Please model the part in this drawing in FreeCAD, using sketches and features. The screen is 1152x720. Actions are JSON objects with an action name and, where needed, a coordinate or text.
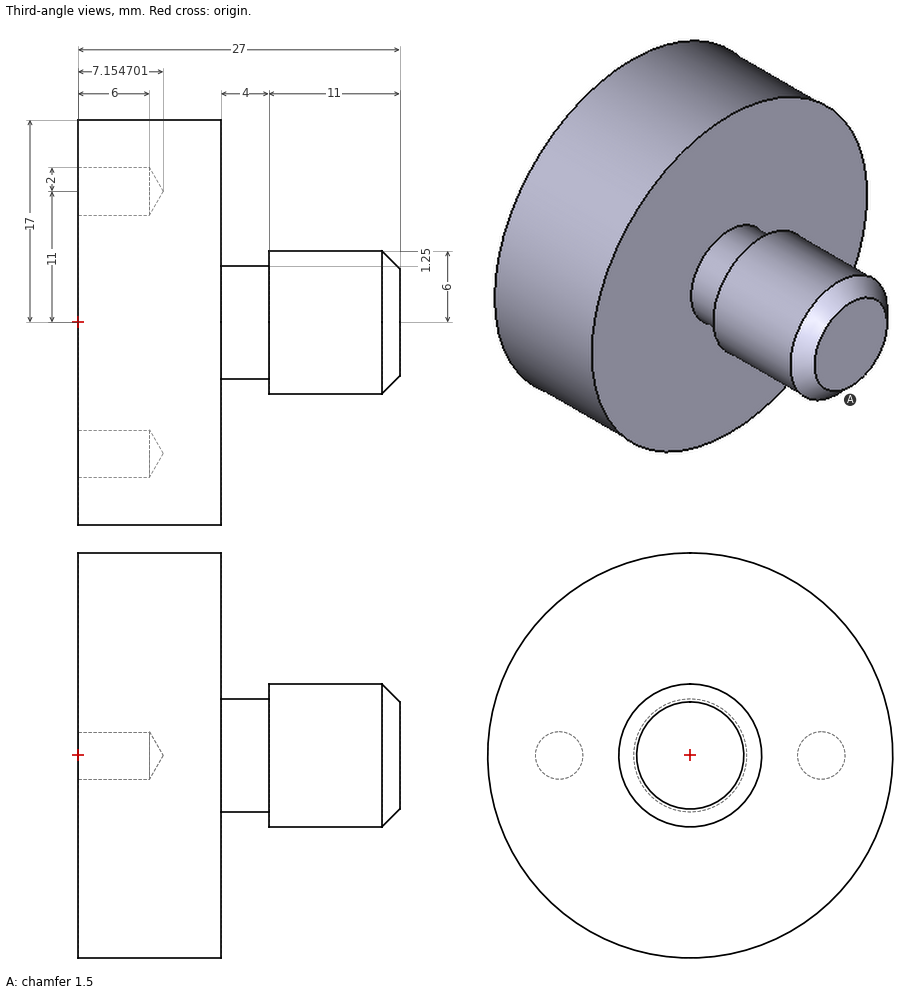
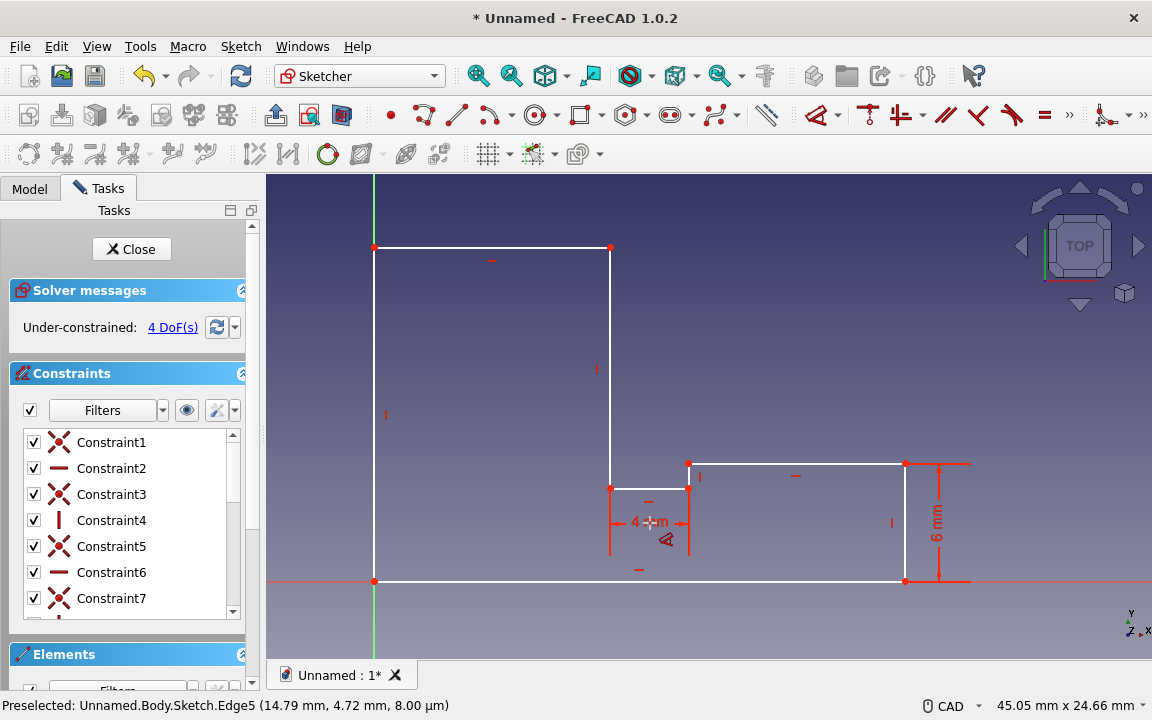
{"action": "left_click", "coordinate": [533, 582]}
{"action": "left_click", "coordinate": [640, 616]}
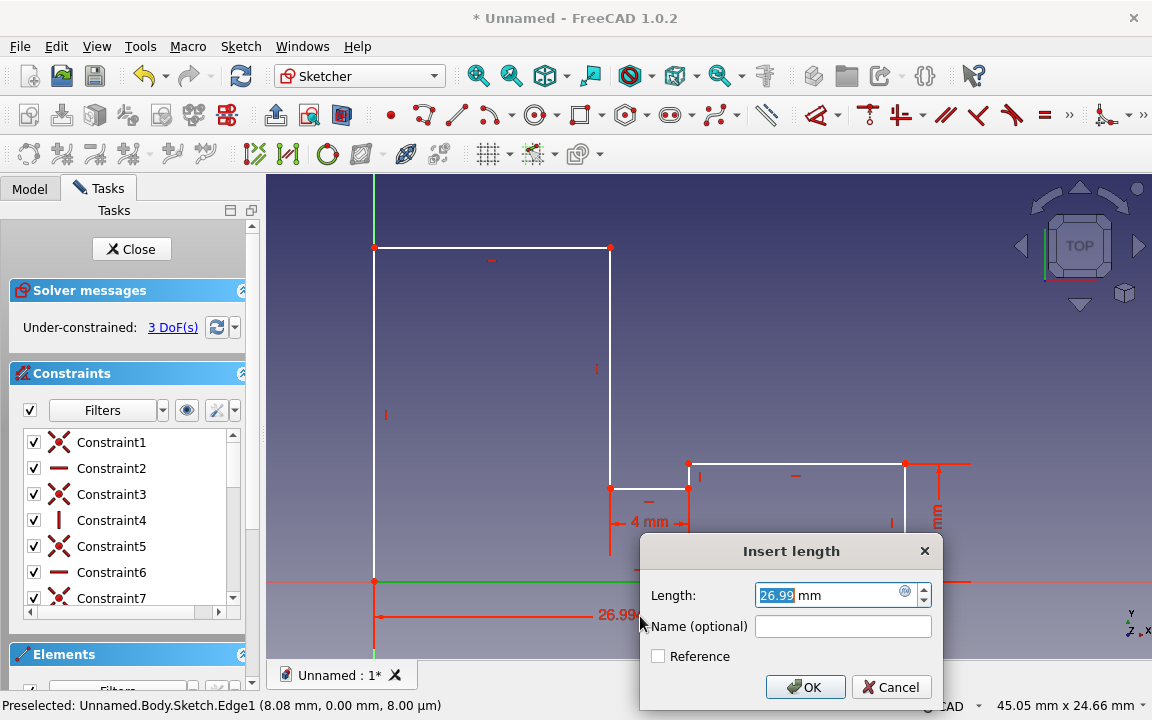
{"action": "type", "text": "27"}
{"action": "key", "text": "Return"}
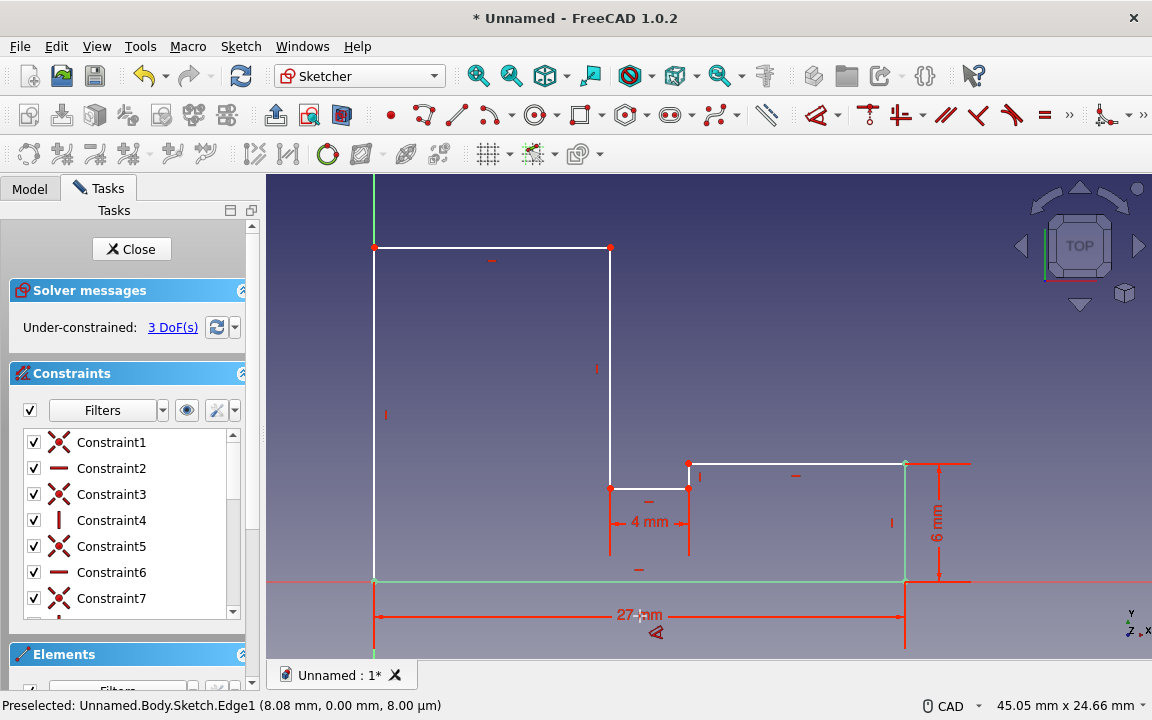
{"action": "left_click", "coordinate": [840, 464]}
{"action": "left_click", "coordinate": [797, 498]}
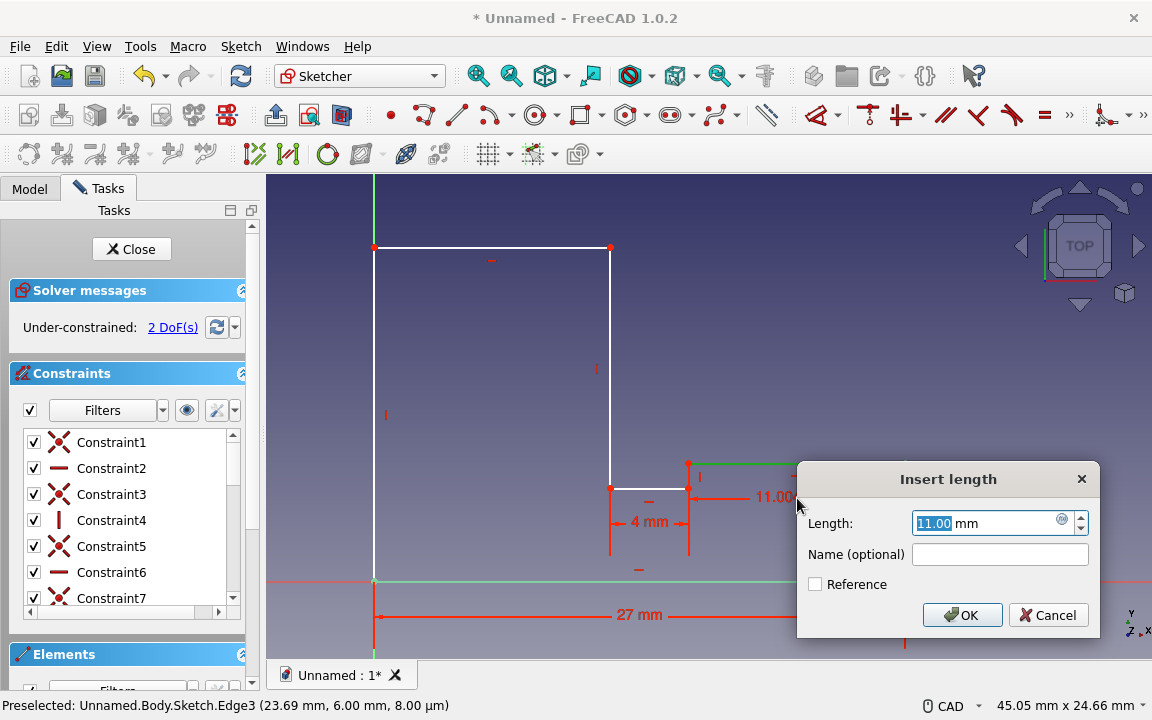
{"action": "type", "text": "11"}
{"action": "key", "text": "Return"}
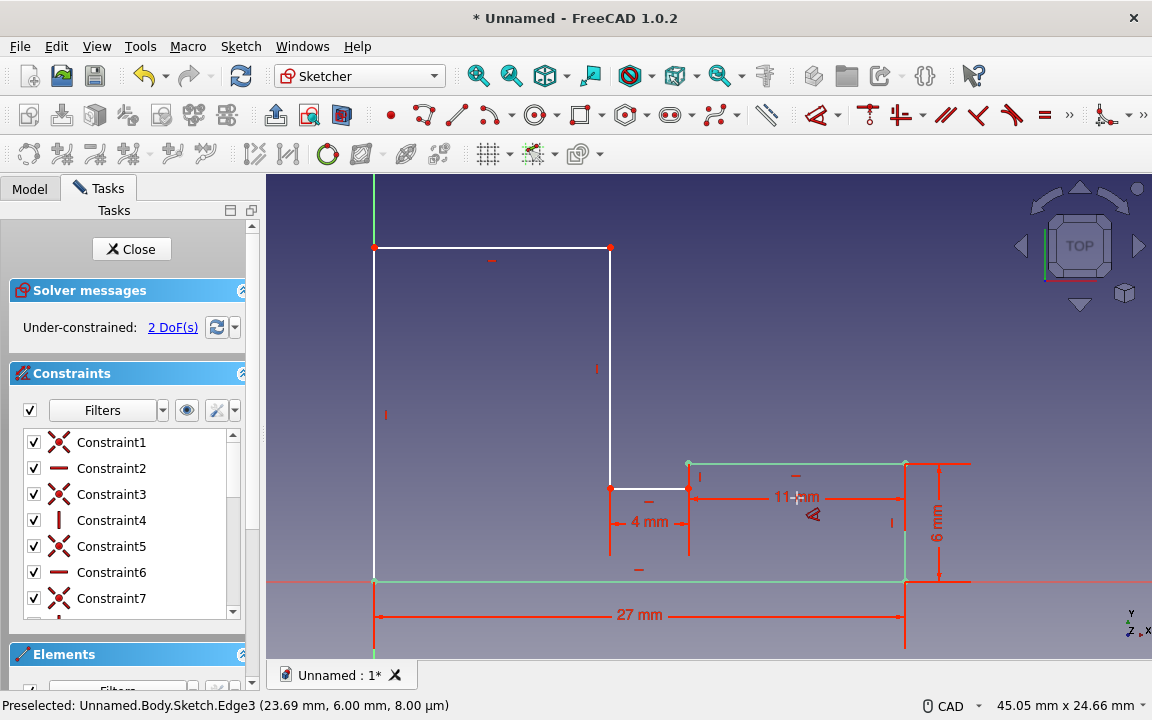
{"action": "left_click", "coordinate": [374, 348]}
{"action": "left_click", "coordinate": [340, 415]}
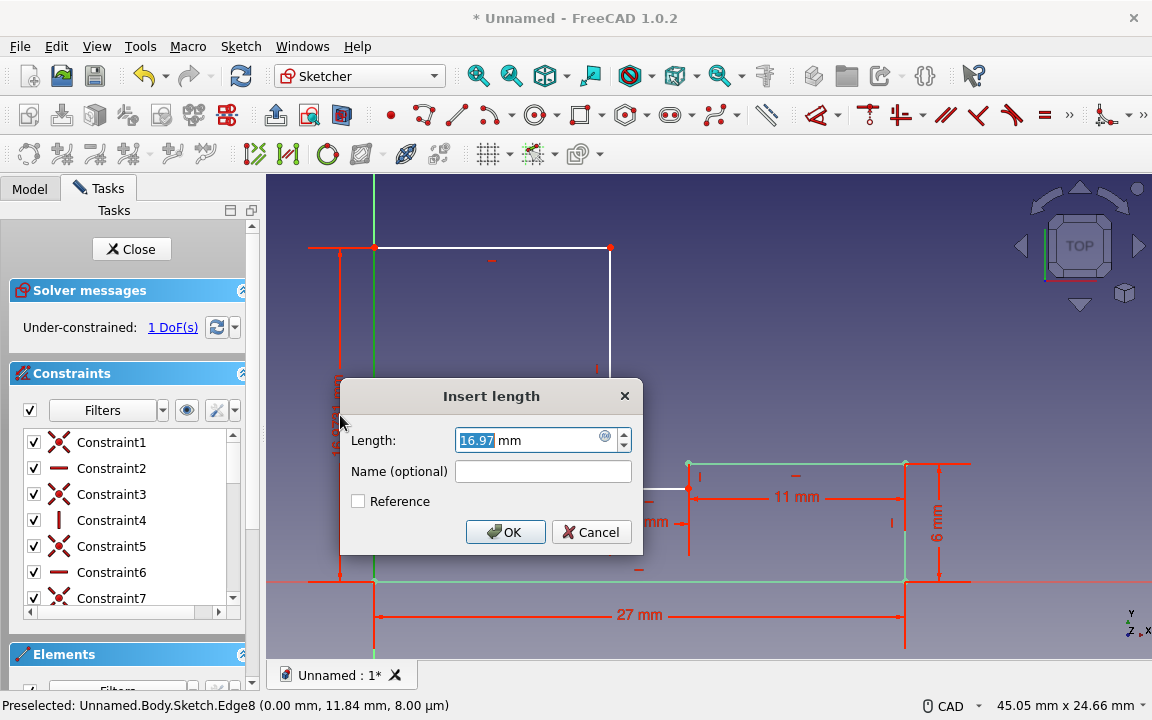
{"action": "type", "text": "17"}
{"action": "key", "text": "Return"}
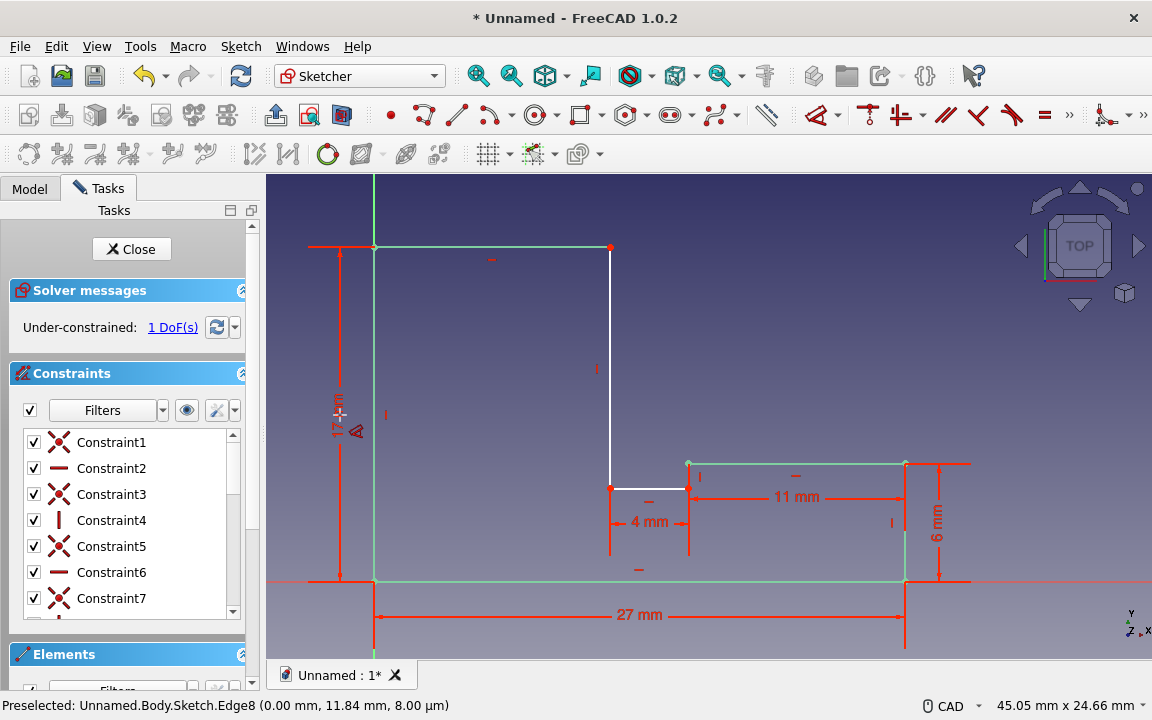
{"action": "scroll", "coordinate": [689, 474], "scroll_direction": "up", "scroll_amount": 3}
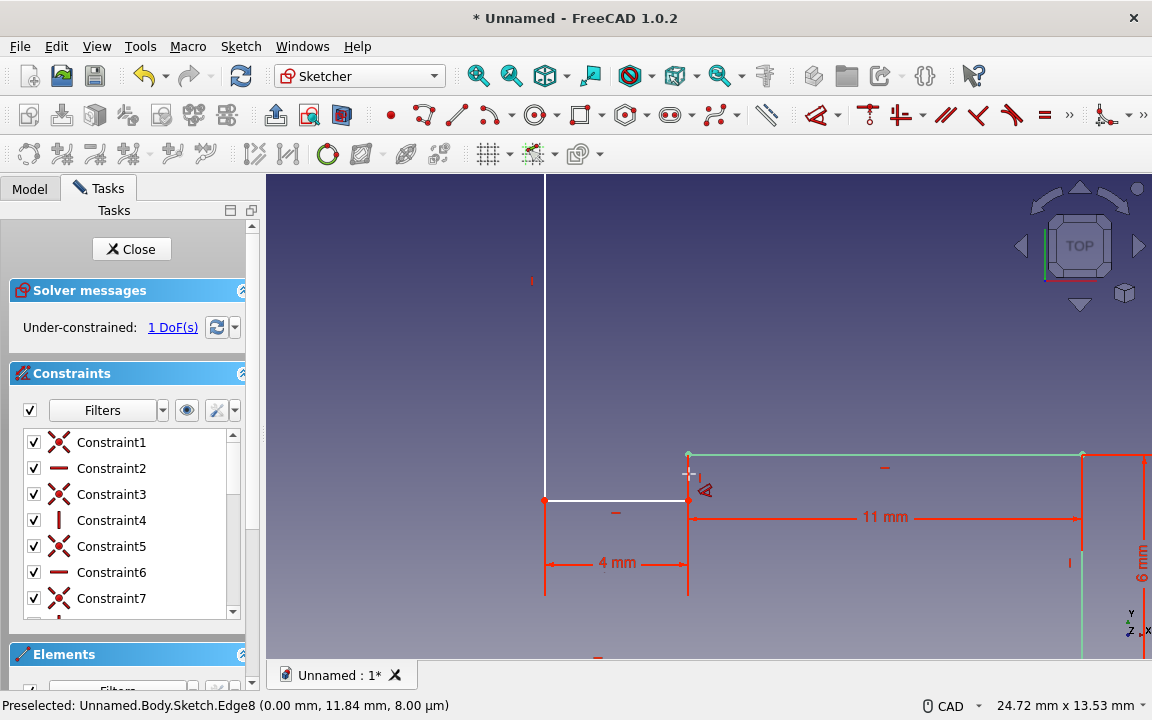
{"action": "left_click", "coordinate": [688, 473]}
{"action": "left_click", "coordinate": [722, 478]}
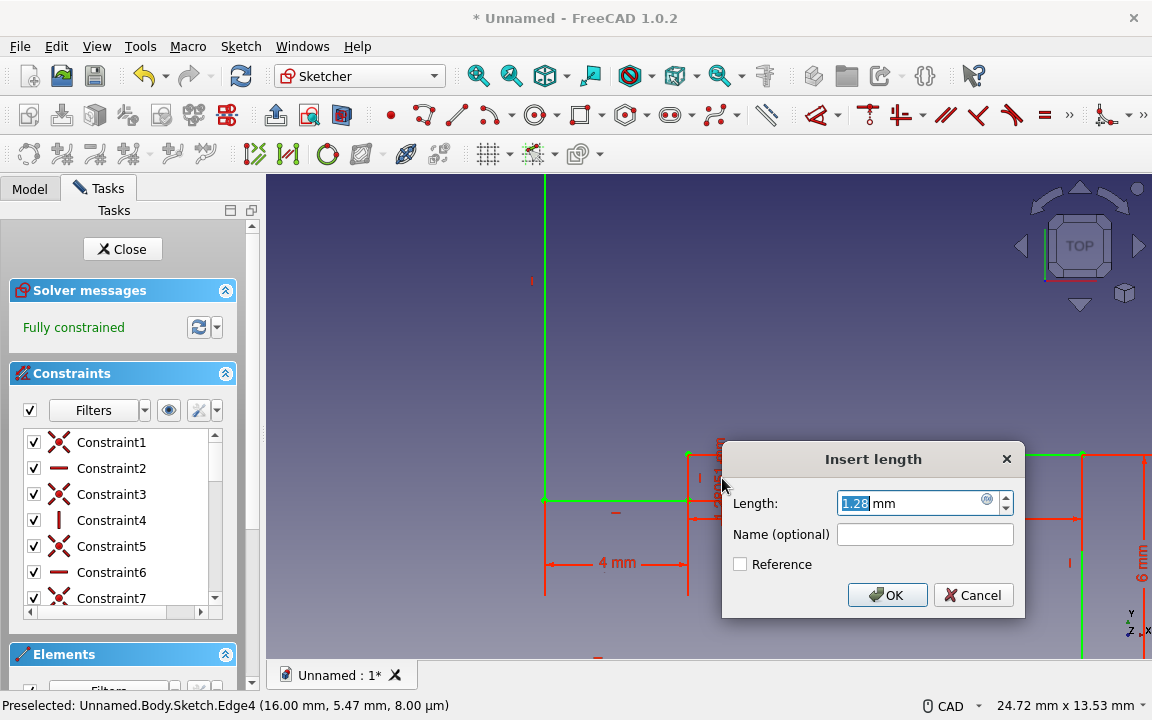
{"action": "type", "text": "1.25"}
{"action": "key", "text": "Return"}
{"action": "key", "text": "Escape"}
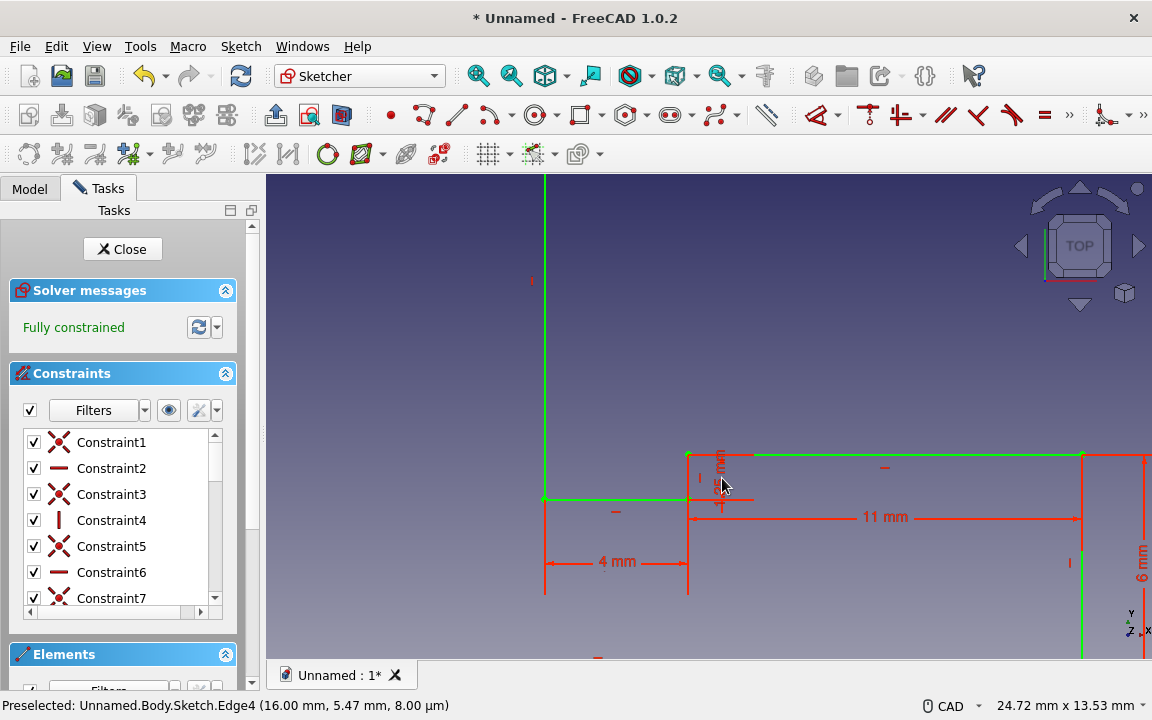
{"action": "left_click", "coordinate": [123, 249]}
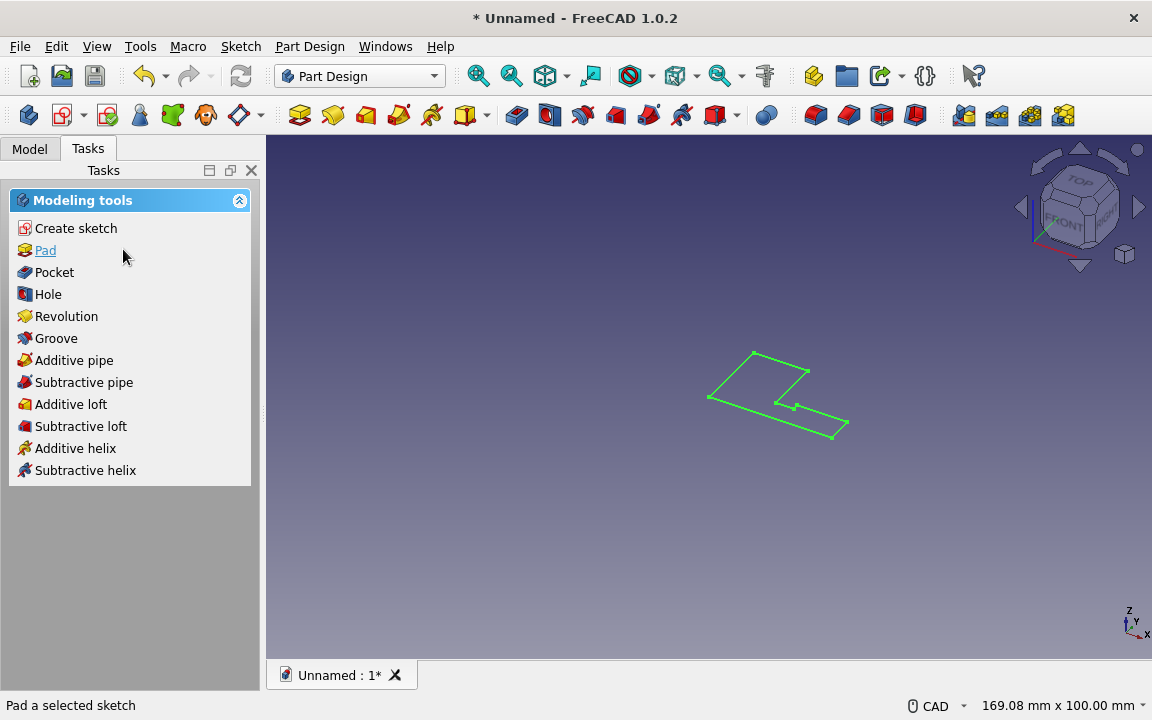
{"action": "left_click", "coordinate": [333, 116]}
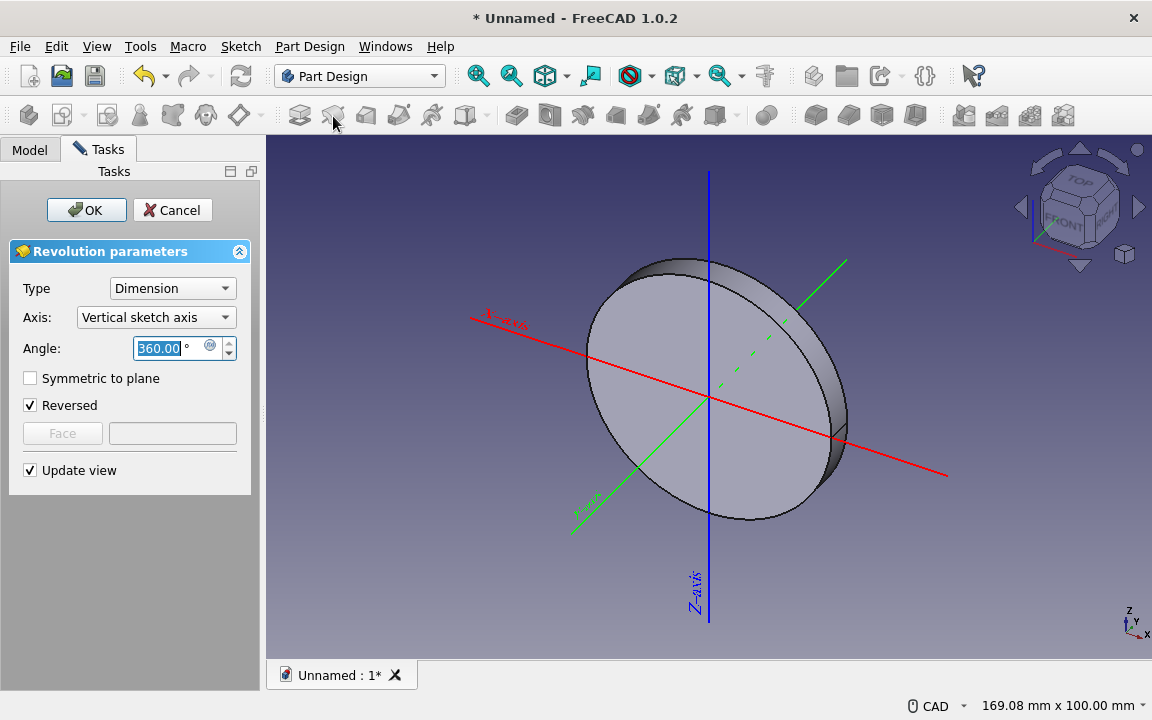
{"action": "left_click", "coordinate": [157, 318]}